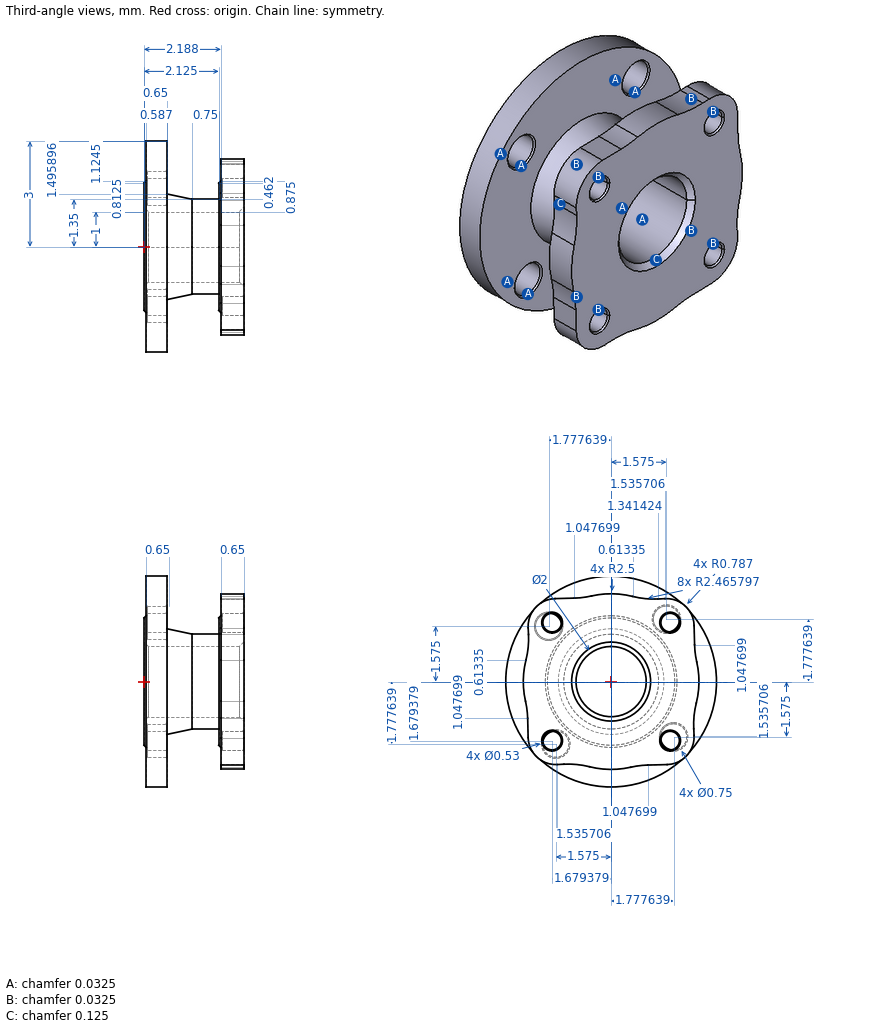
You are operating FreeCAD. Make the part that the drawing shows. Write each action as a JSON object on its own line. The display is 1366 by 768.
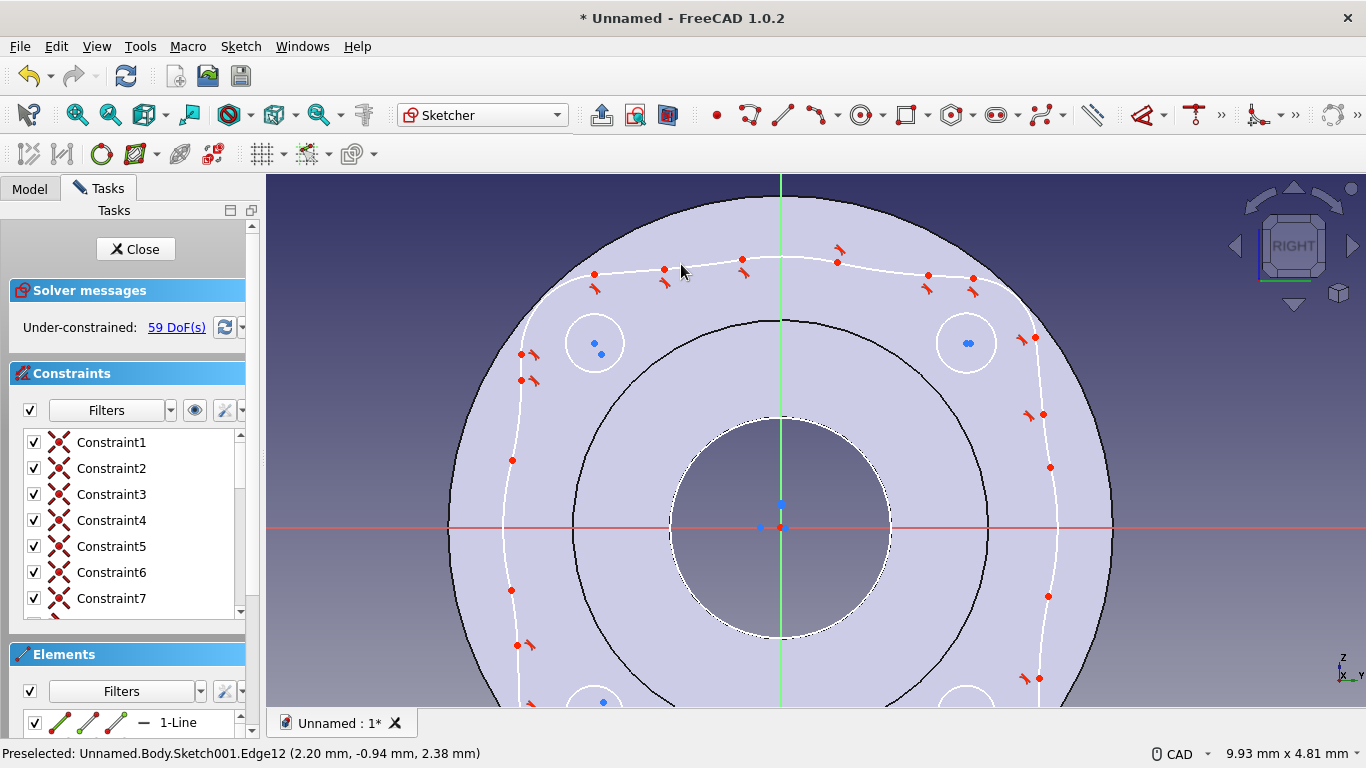
{"action": "left_click", "coordinate": [517, 437]}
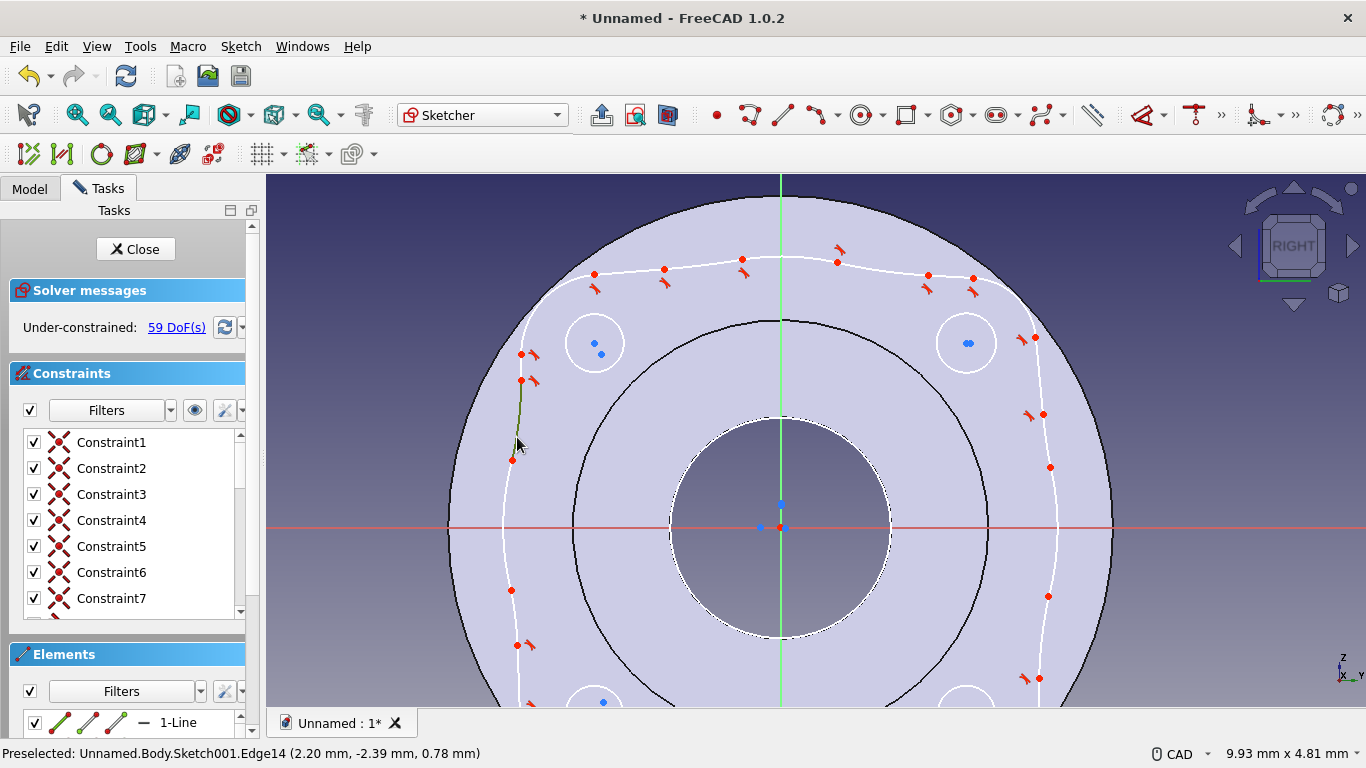
{"action": "left_click", "coordinate": [505, 500]}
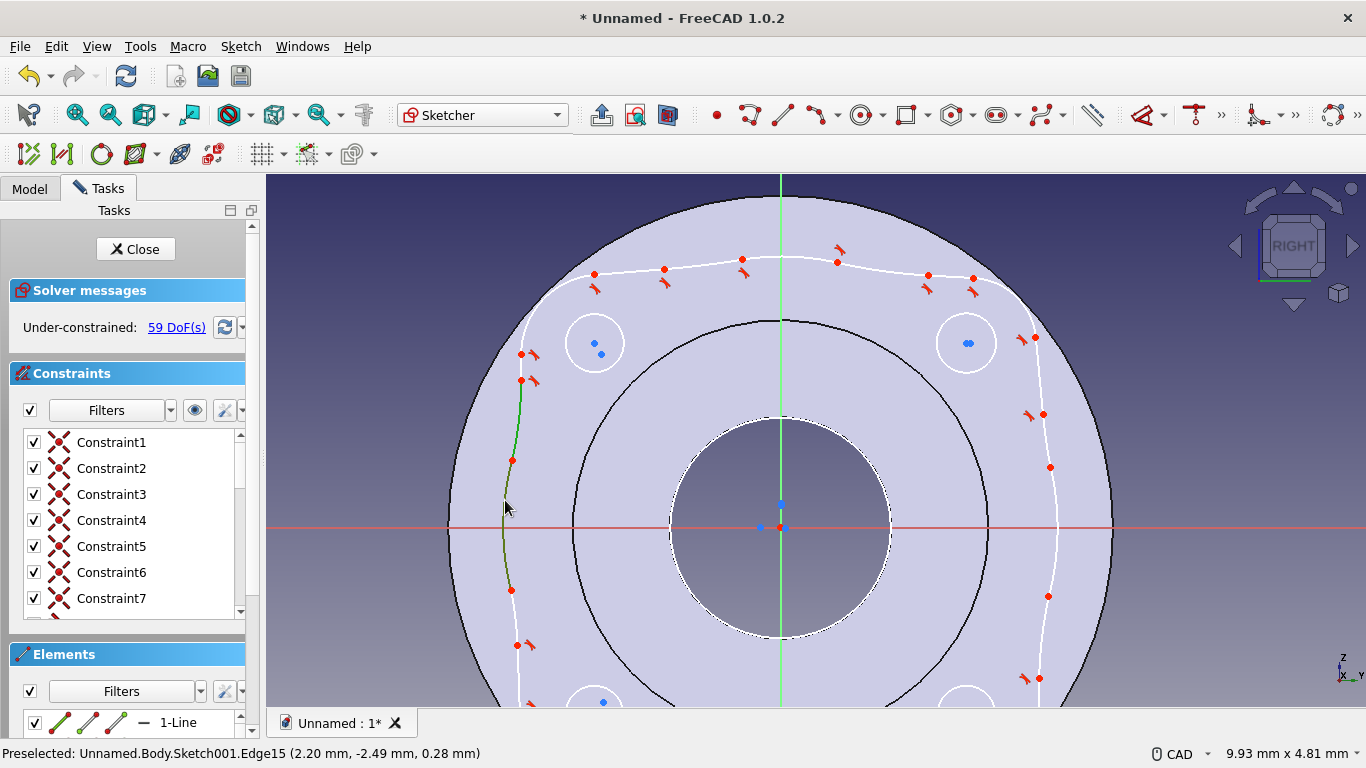
{"action": "key", "text": "t"}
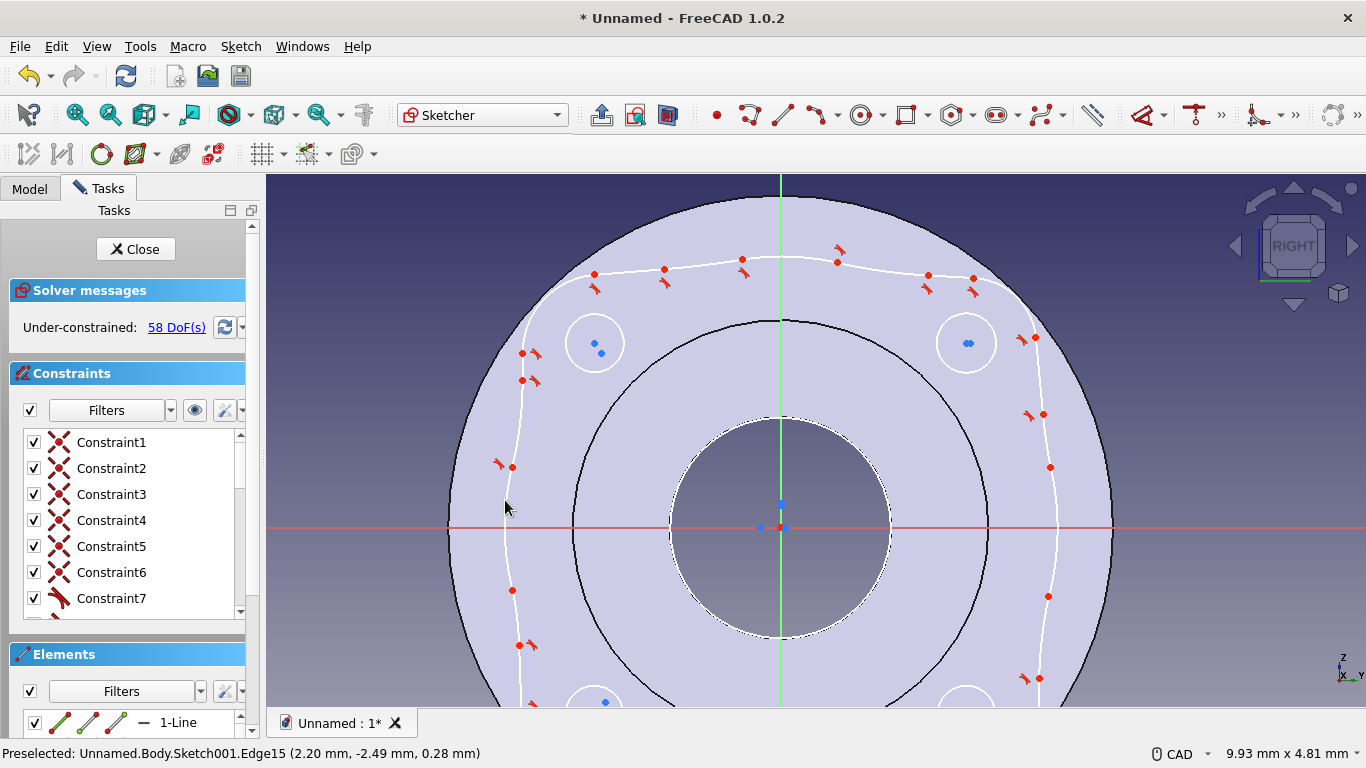
{"action": "left_click", "coordinate": [506, 504]}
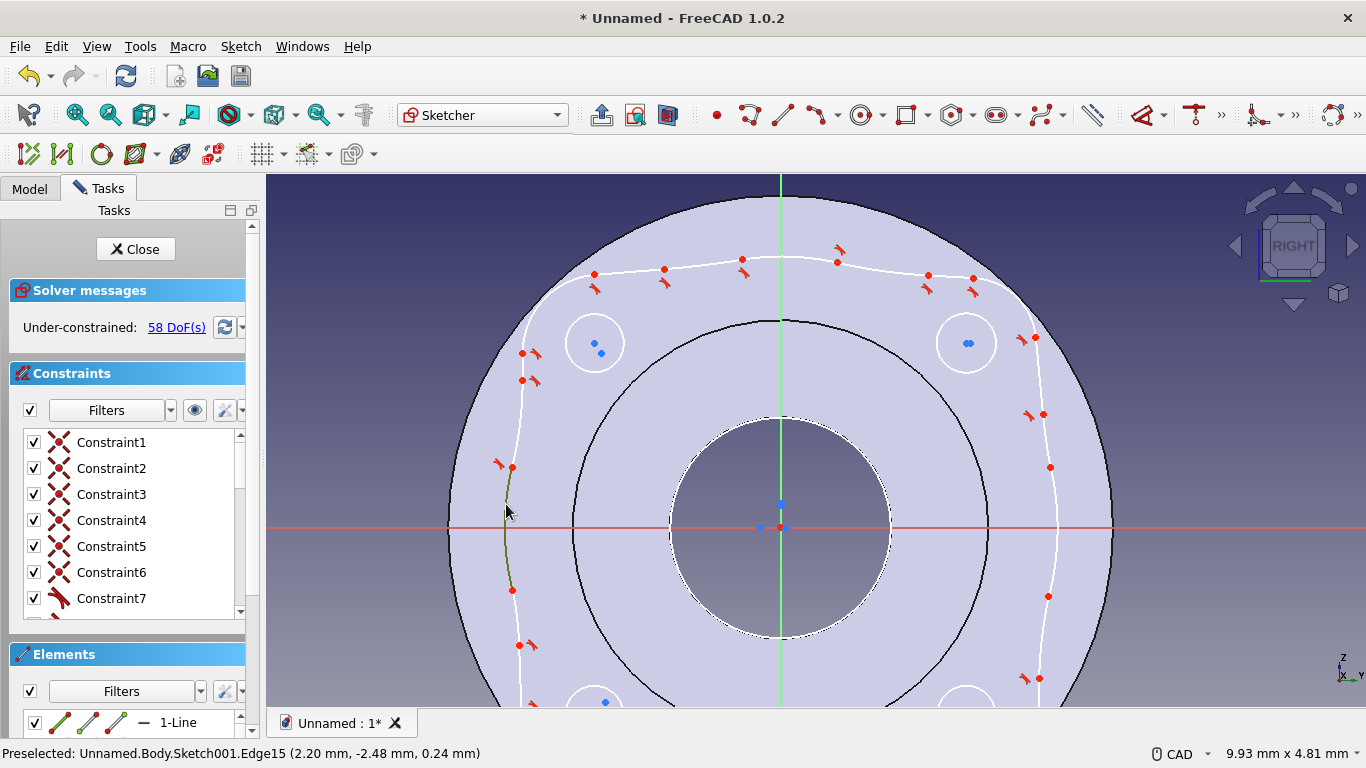
{"action": "left_click", "coordinate": [518, 629]}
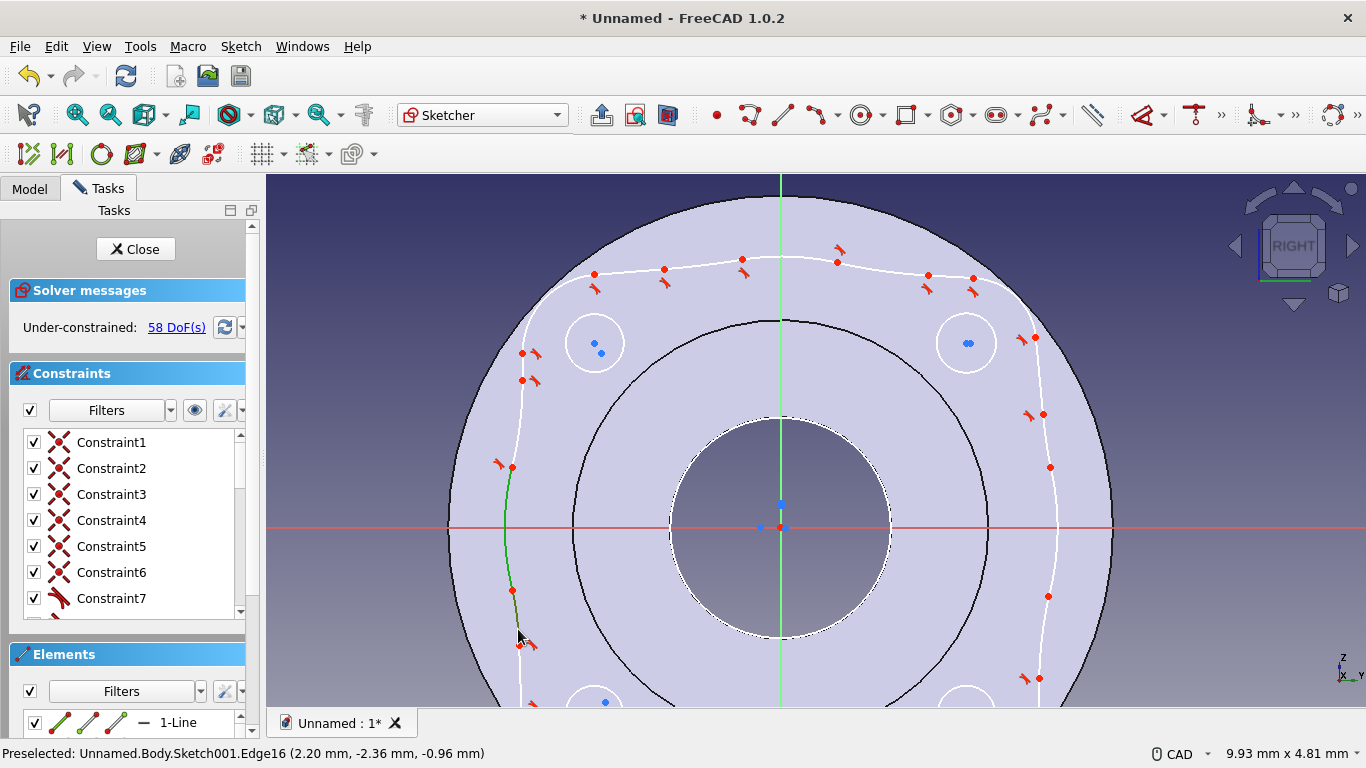
{"action": "key", "text": "t"}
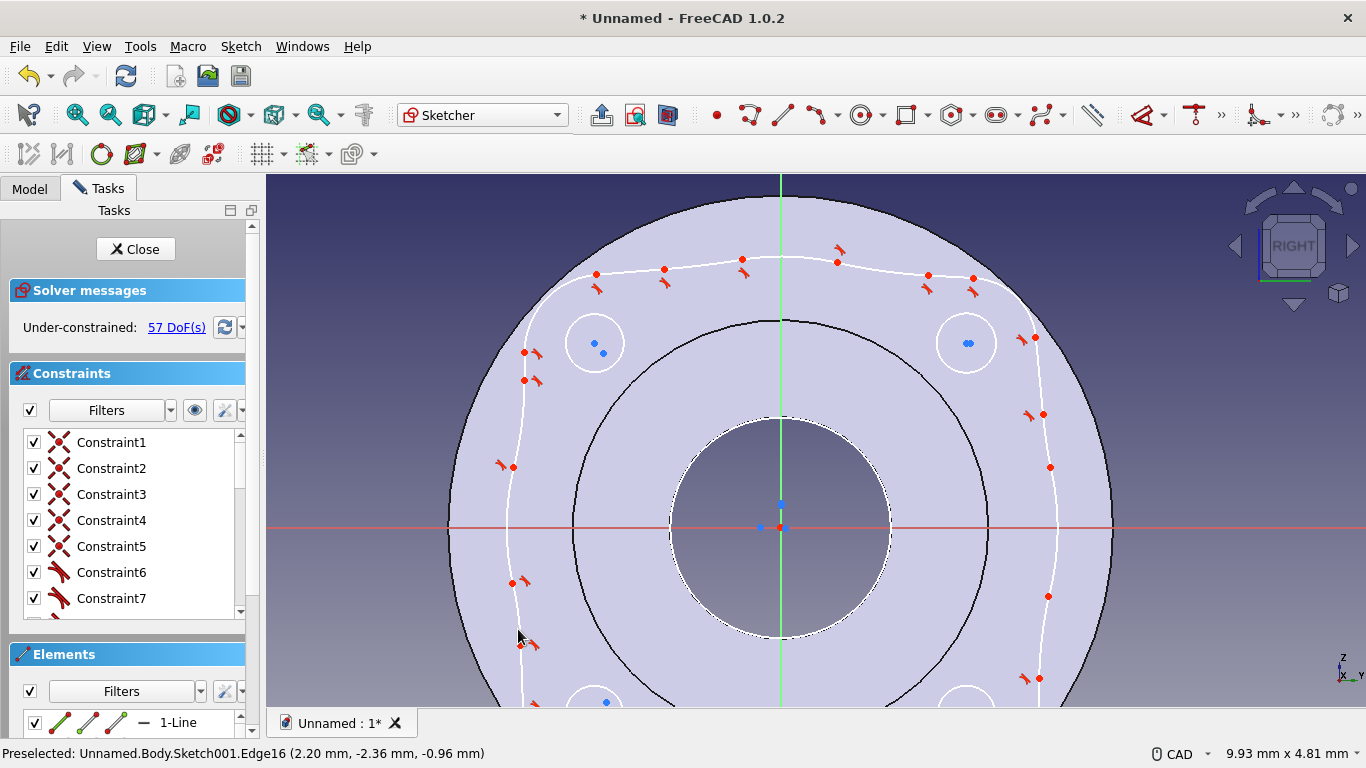
{"action": "scroll", "coordinate": [680, 263], "scroll_direction": "down", "scroll_amount": 2}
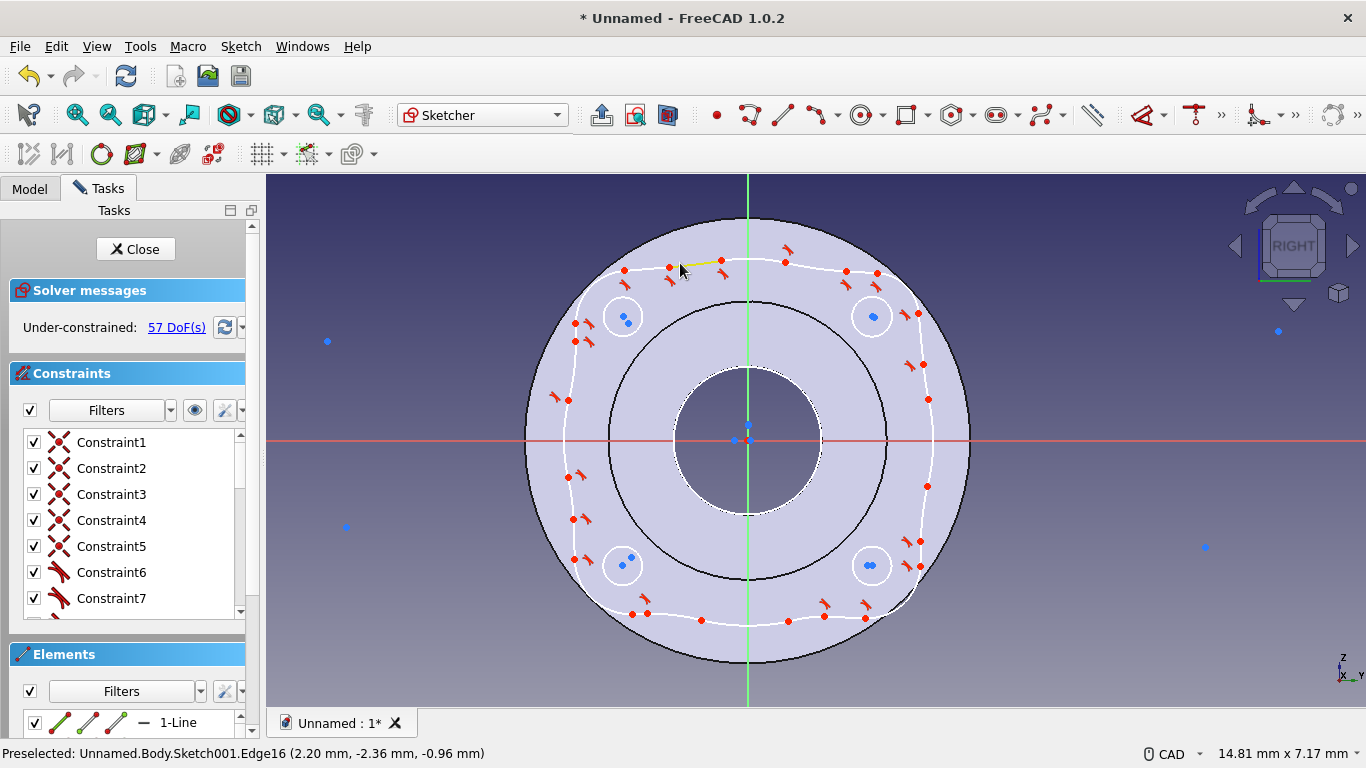
{"action": "left_click", "coordinate": [686, 617]}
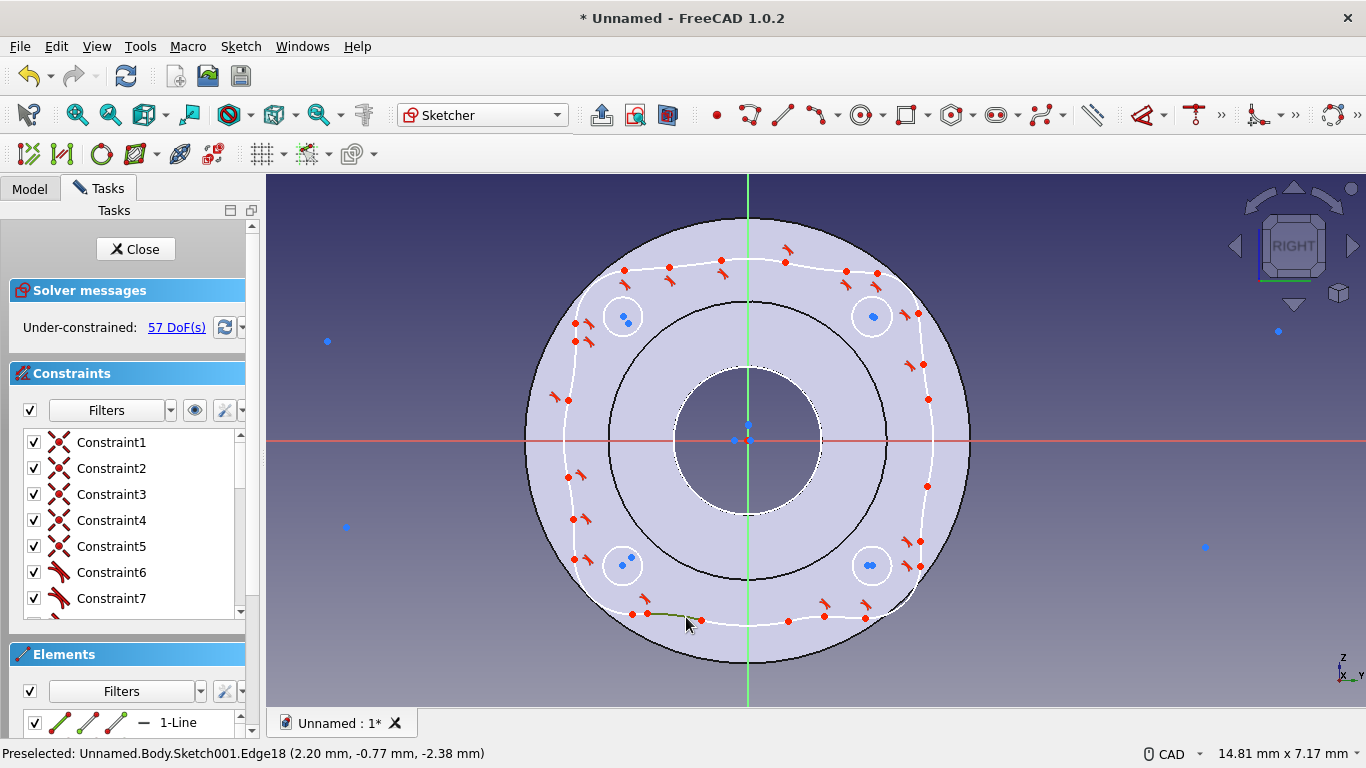
{"action": "left_click", "coordinate": [728, 625]}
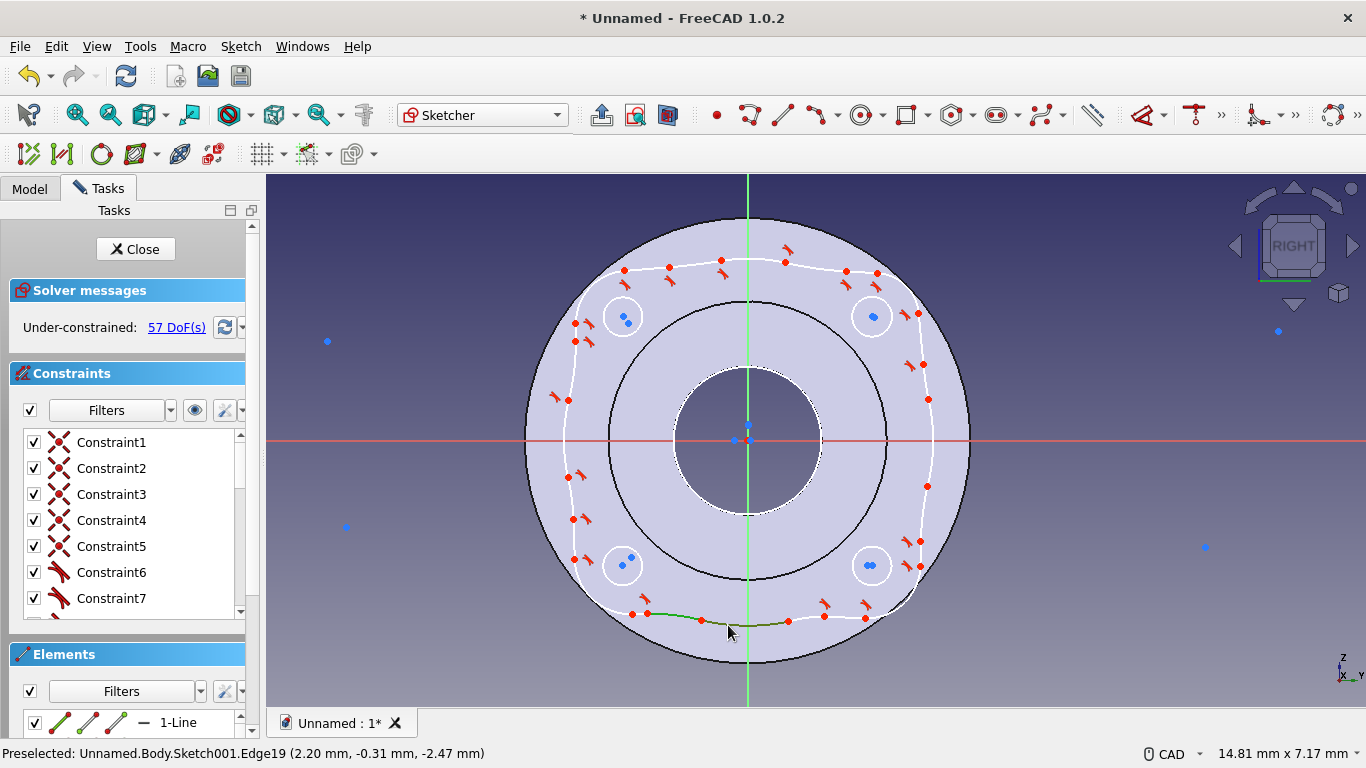
{"action": "key", "text": "t"}